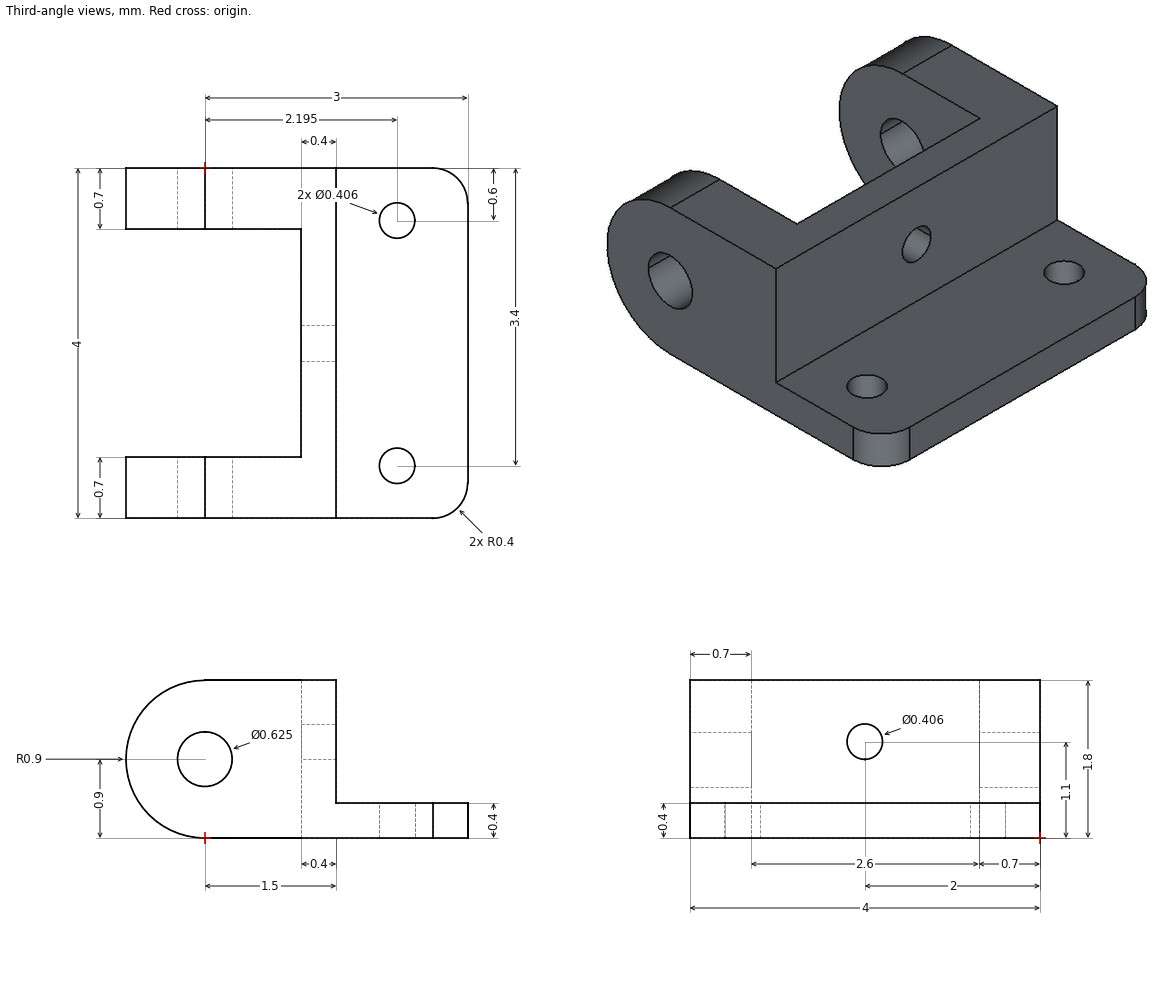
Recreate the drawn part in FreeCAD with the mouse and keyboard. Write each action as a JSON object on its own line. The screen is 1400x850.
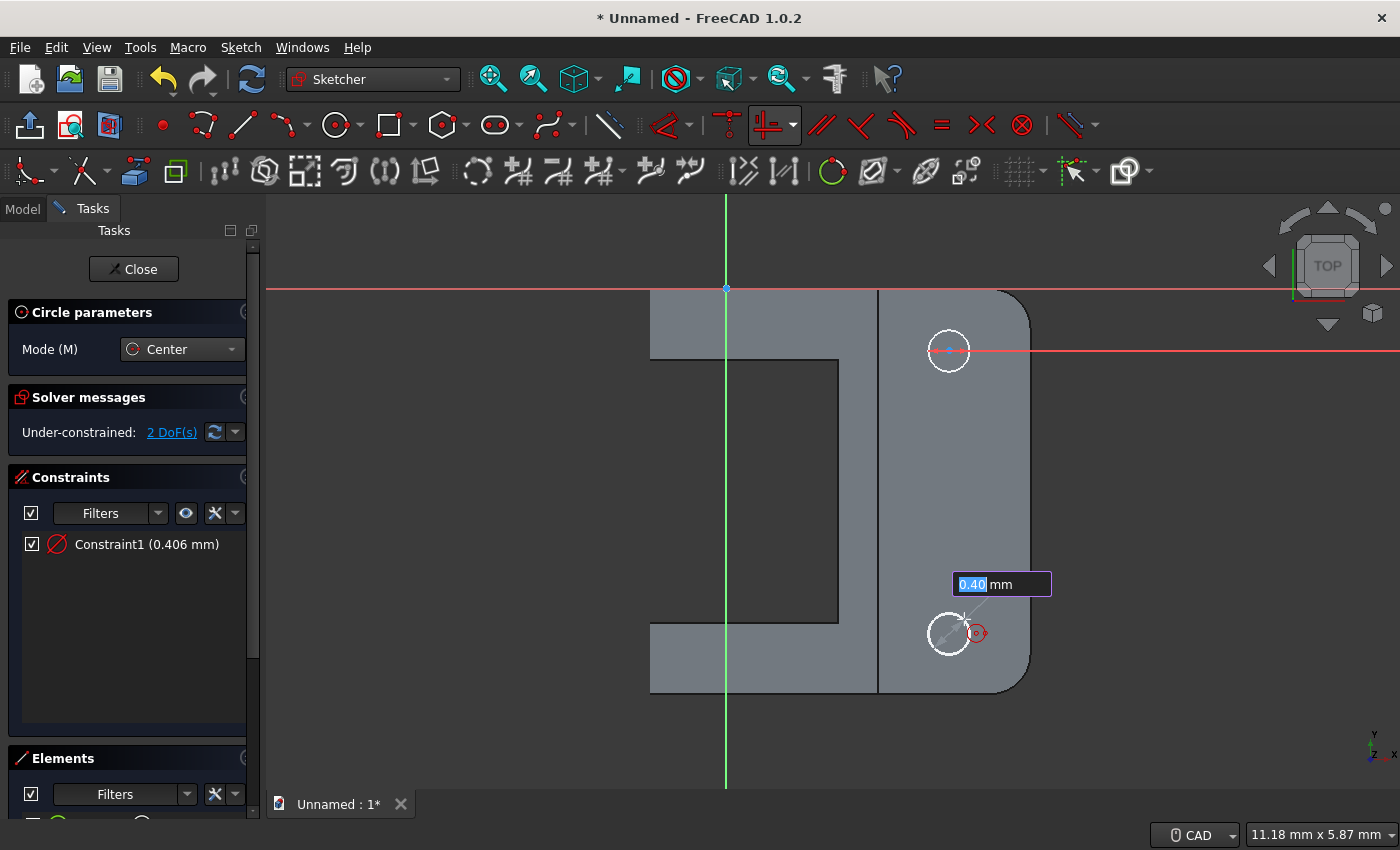
{"action": "type", "text": "0.406"}
{"action": "key", "text": "Return"}
{"action": "key", "text": "Escape"}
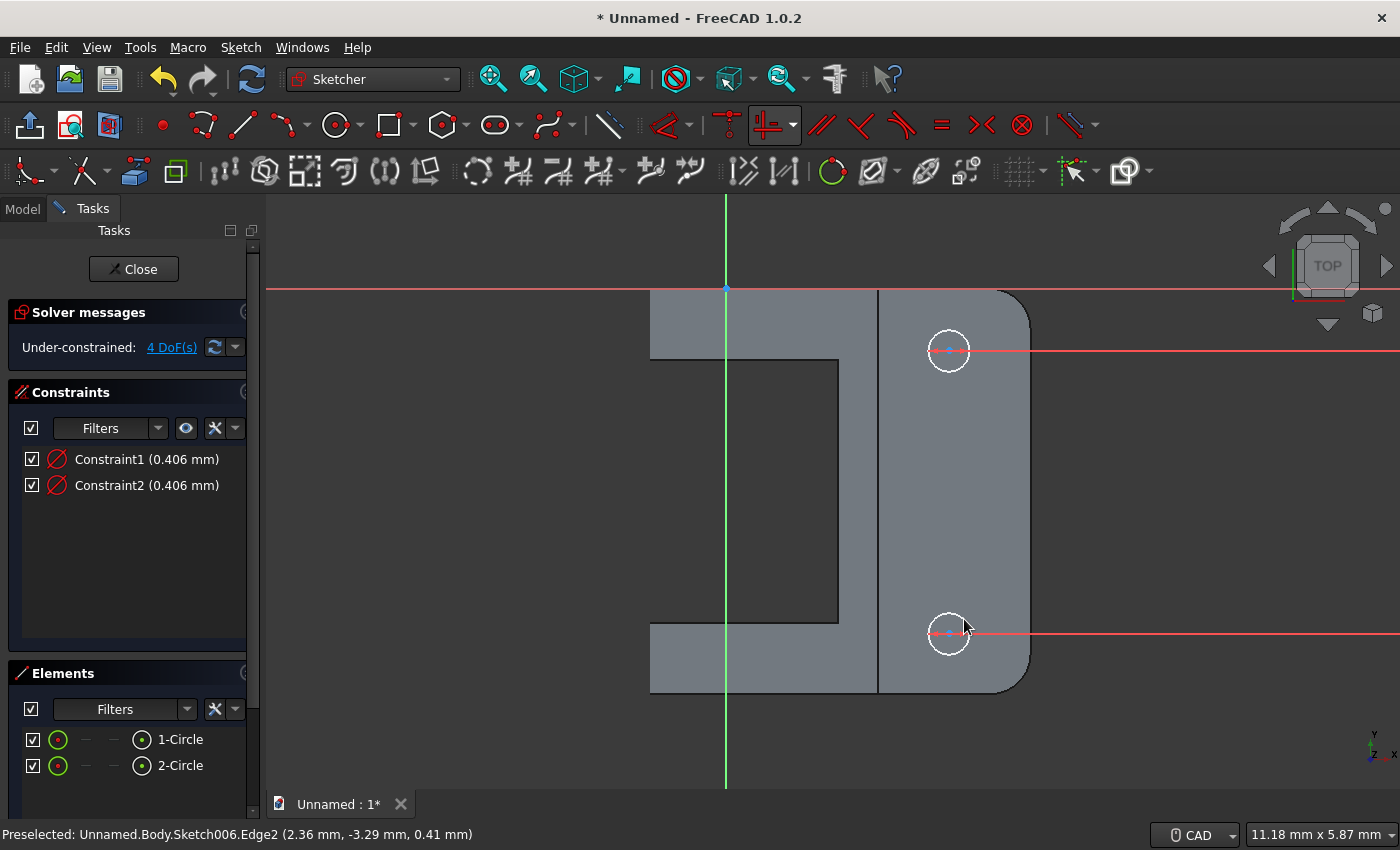
{"action": "left_click", "coordinate": [949, 351]}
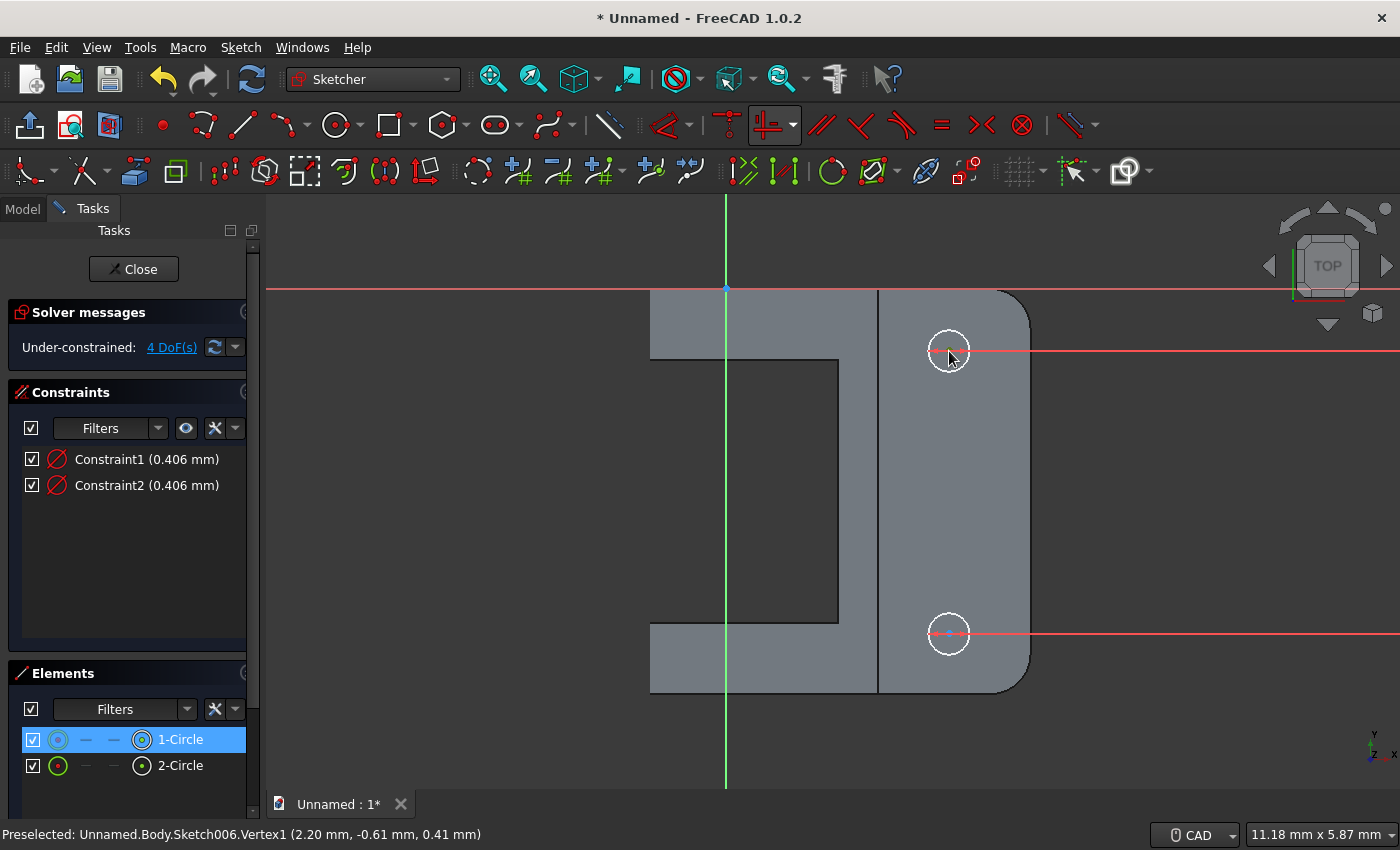
{"action": "left_click", "coordinate": [949, 634]}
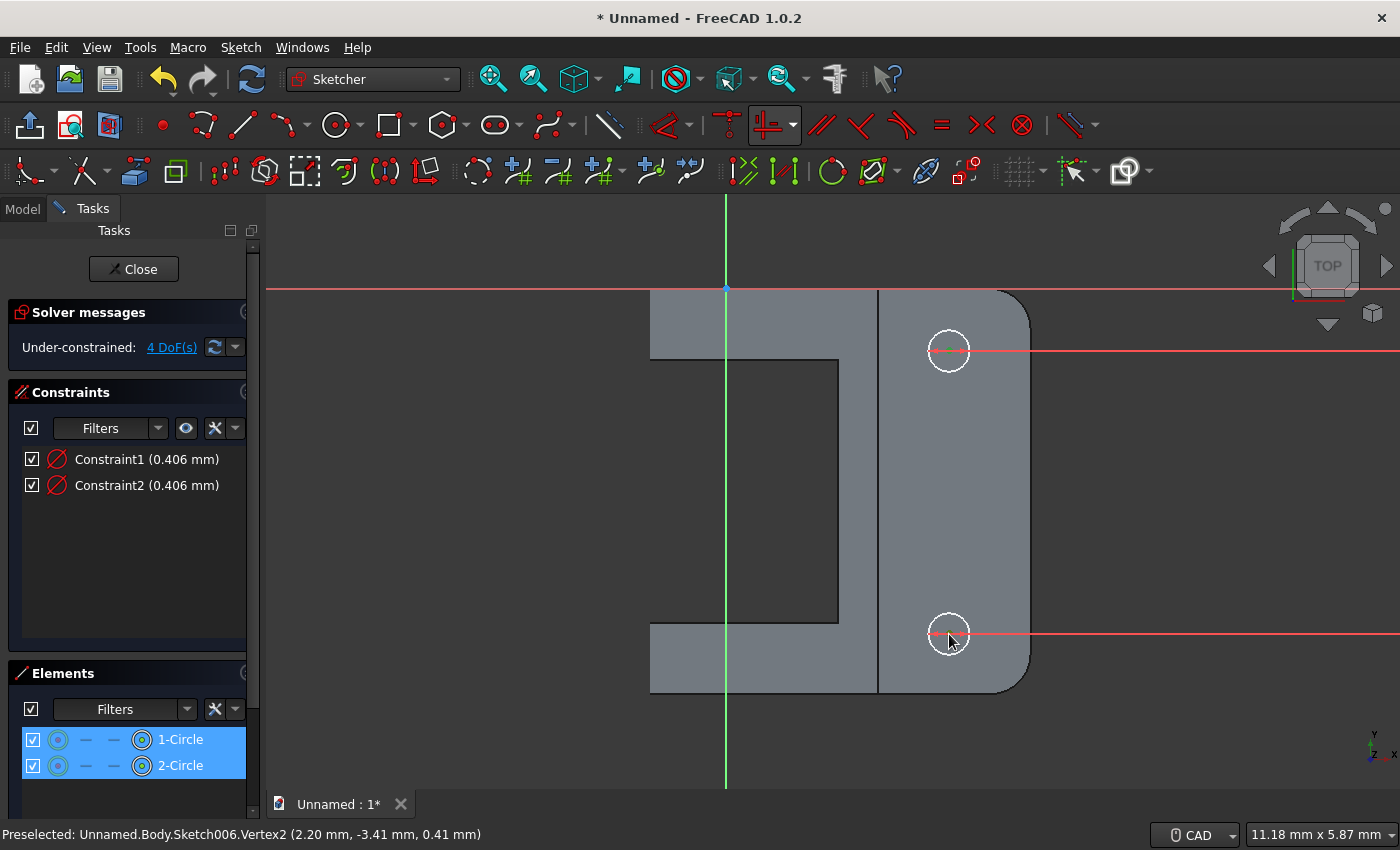
{"action": "key", "text": "v"}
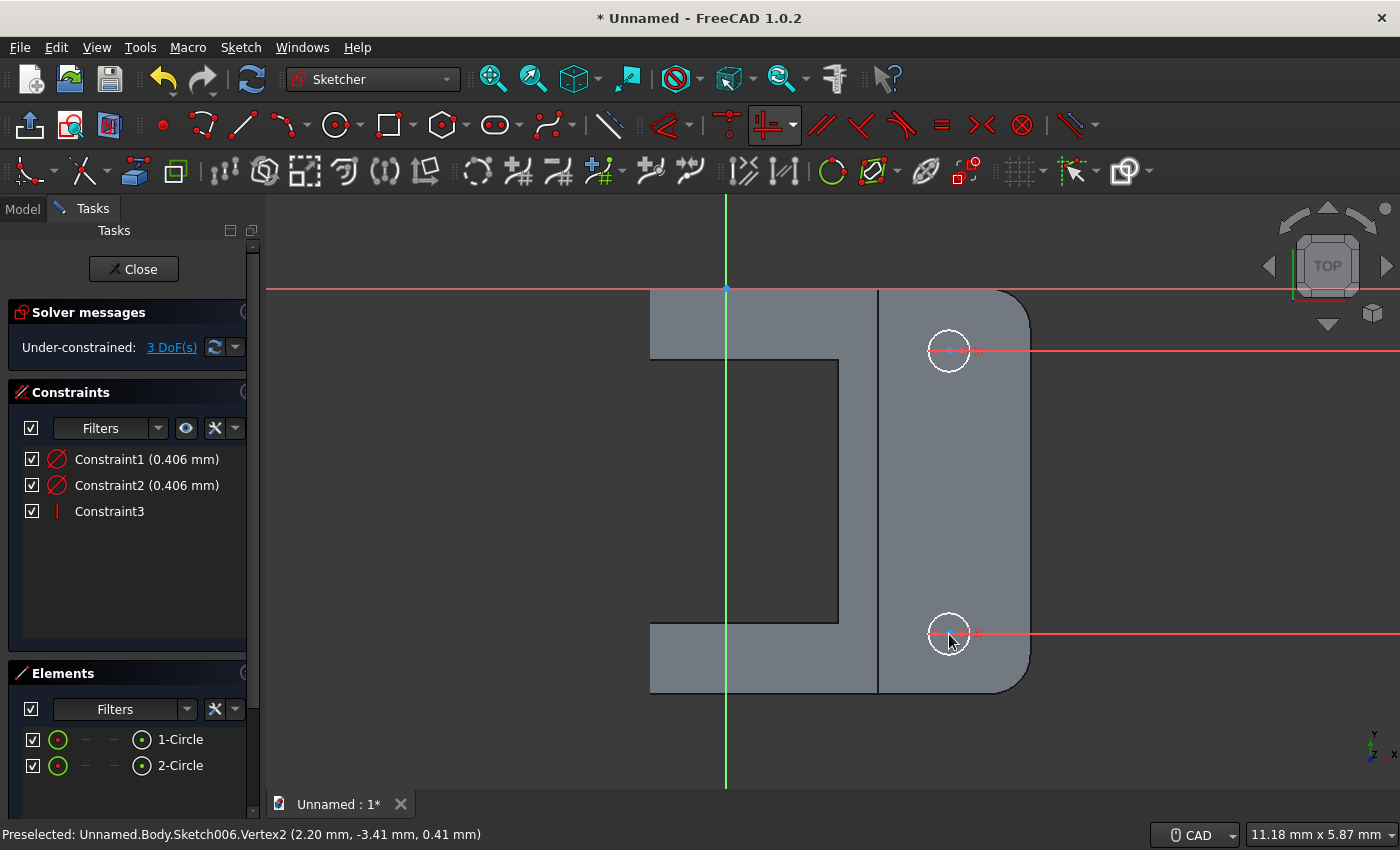
{"action": "left_click", "coordinate": [664, 126]}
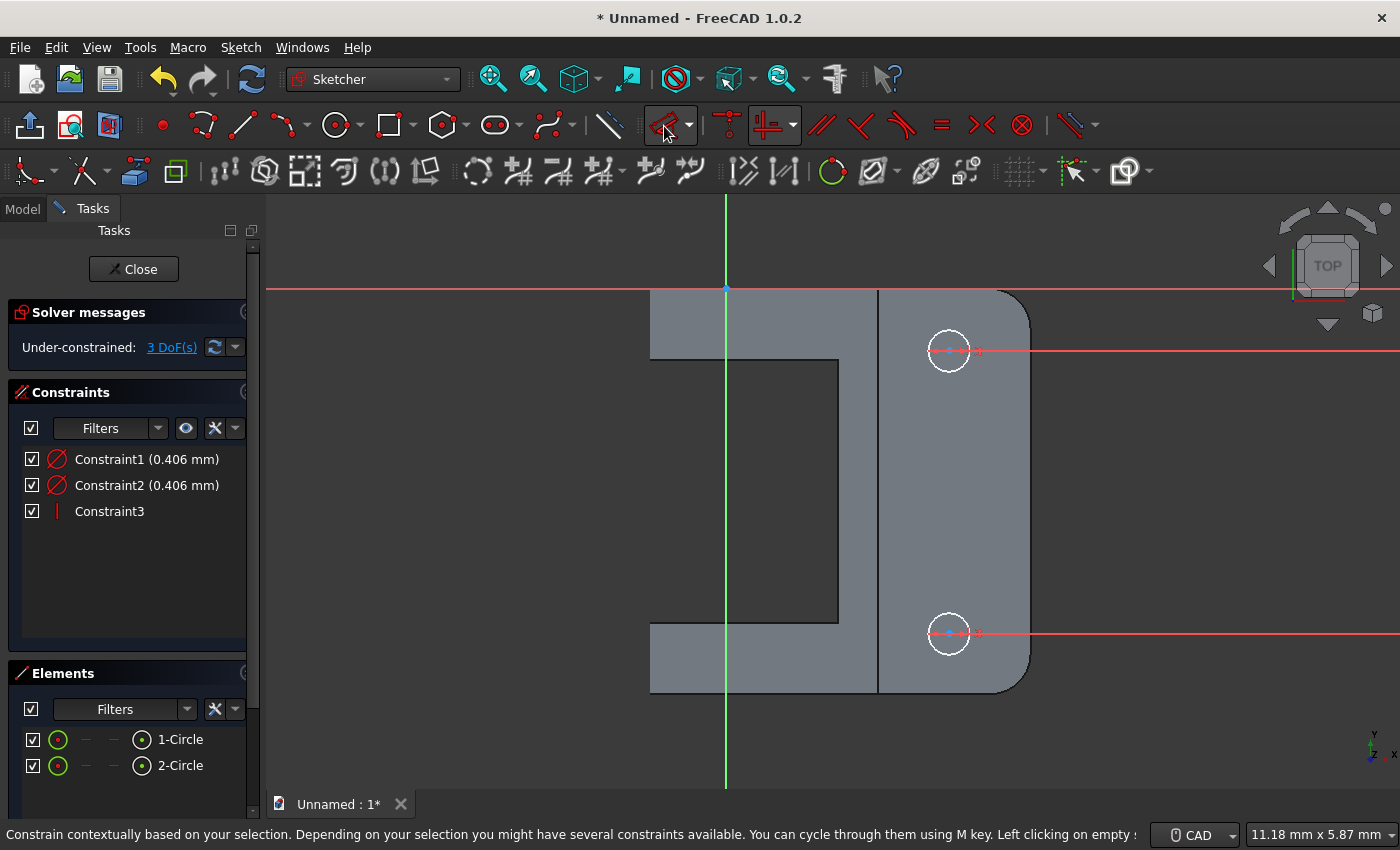
{"action": "left_click", "coordinate": [949, 351]}
{"action": "left_click", "coordinate": [692, 320]}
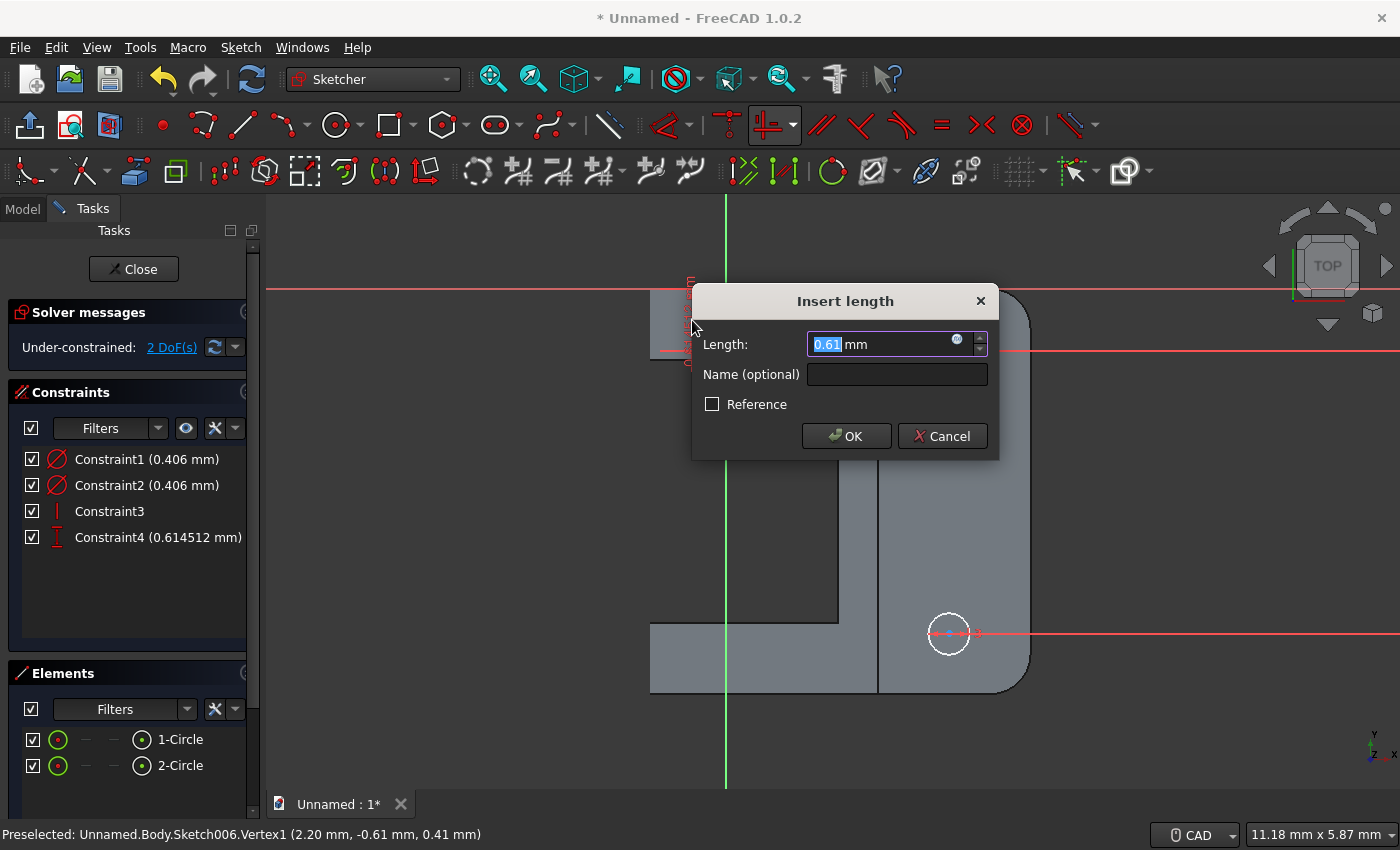
{"action": "type", "text": "0.6"}
{"action": "key", "text": "Return"}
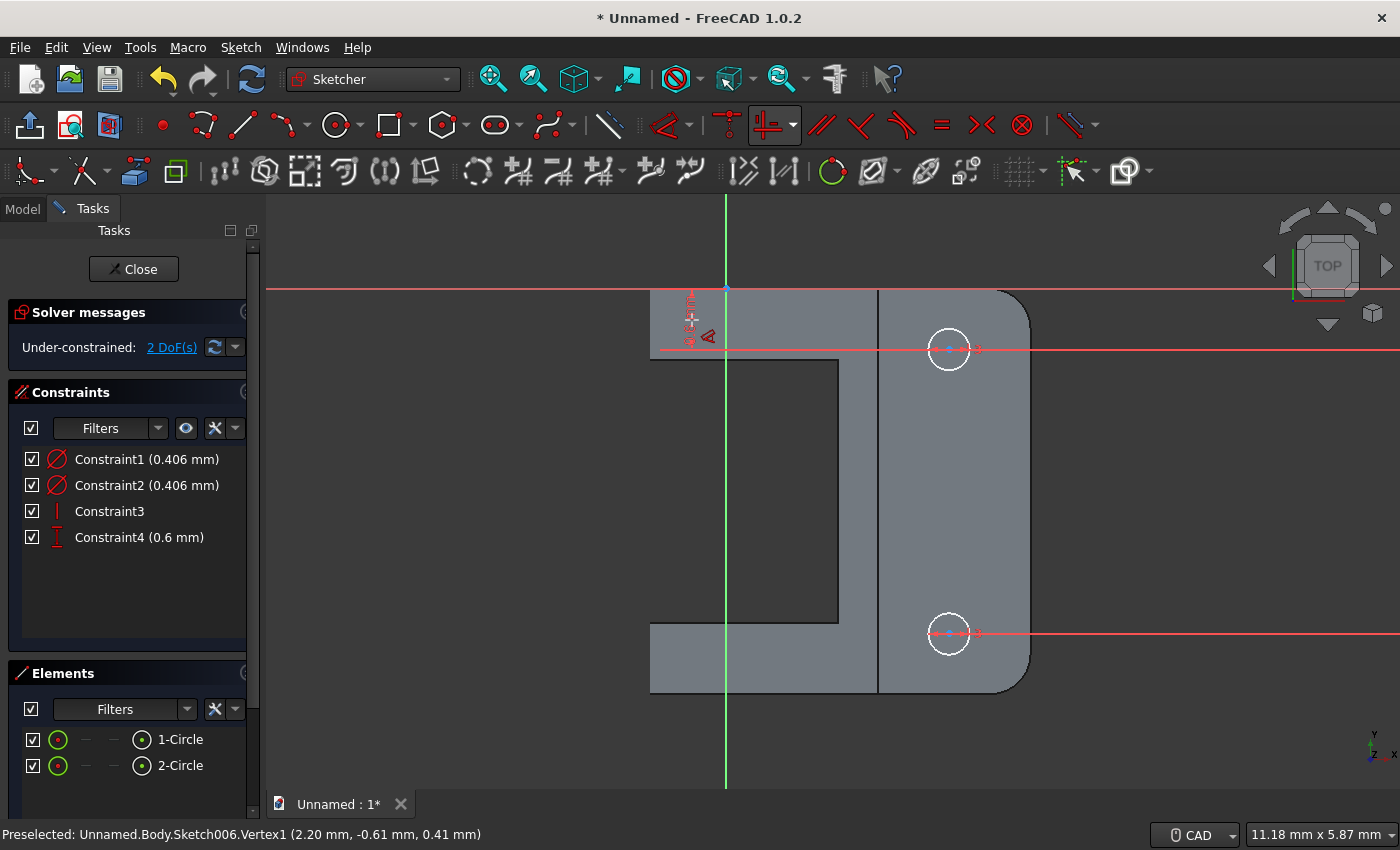
{"action": "left_click", "coordinate": [949, 634]}
{"action": "left_click", "coordinate": [692, 461]}